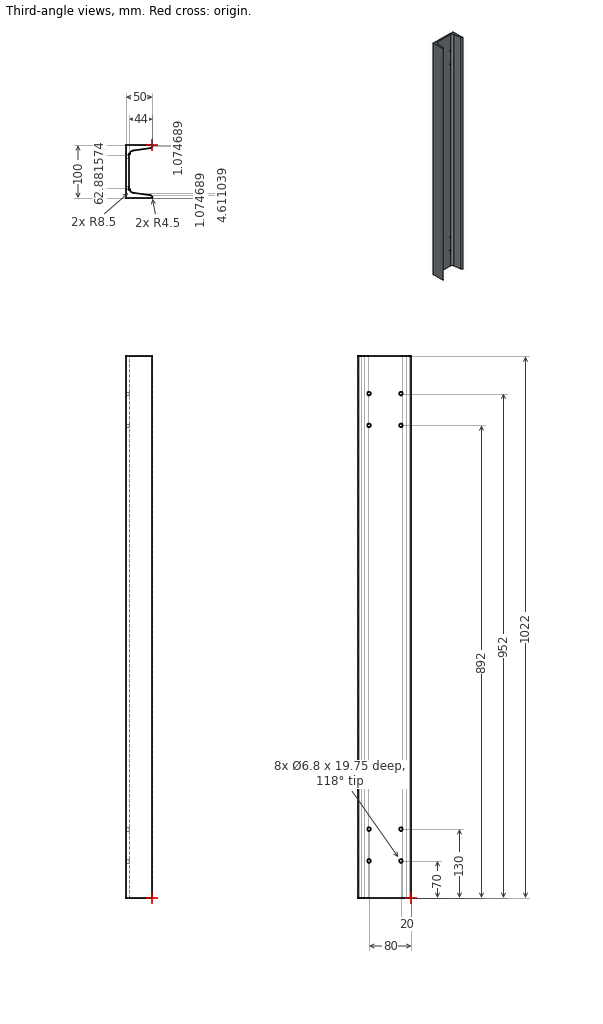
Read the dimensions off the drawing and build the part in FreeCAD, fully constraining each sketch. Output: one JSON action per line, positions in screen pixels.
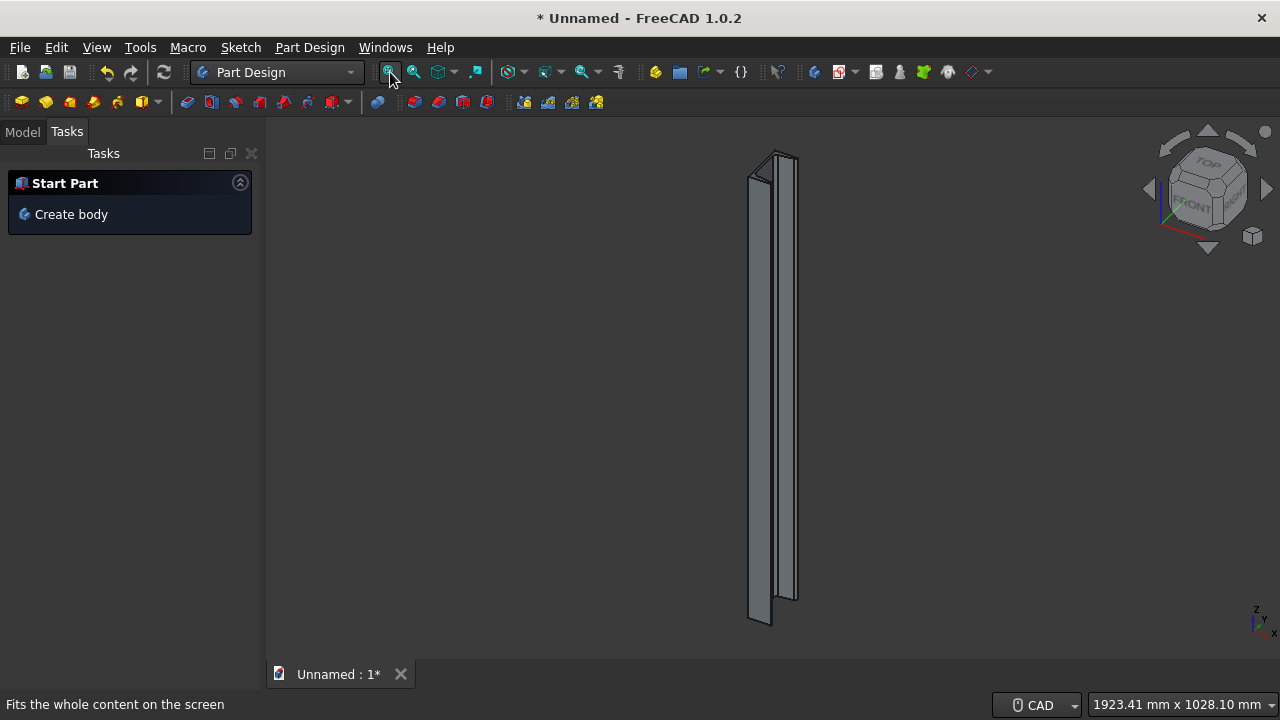
{"action": "key", "text": "6"}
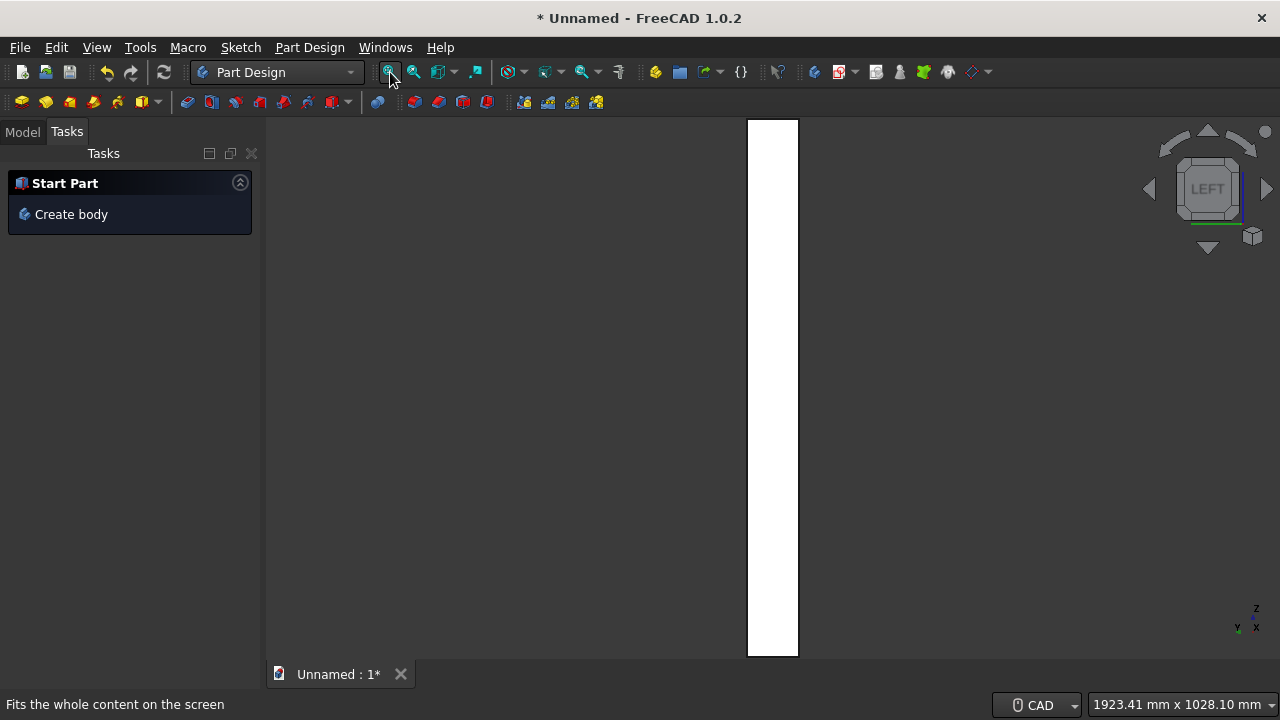
{"action": "left_click", "coordinate": [773, 156]}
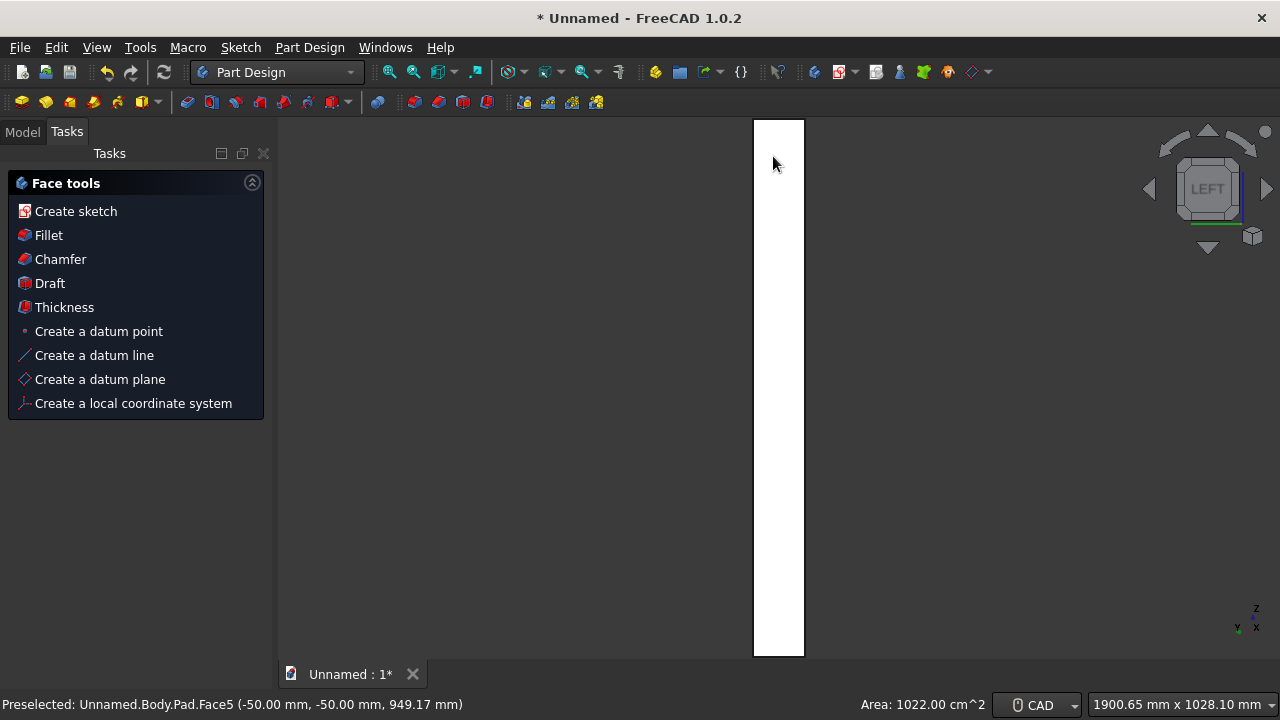
{"action": "left_click", "coordinate": [840, 72]}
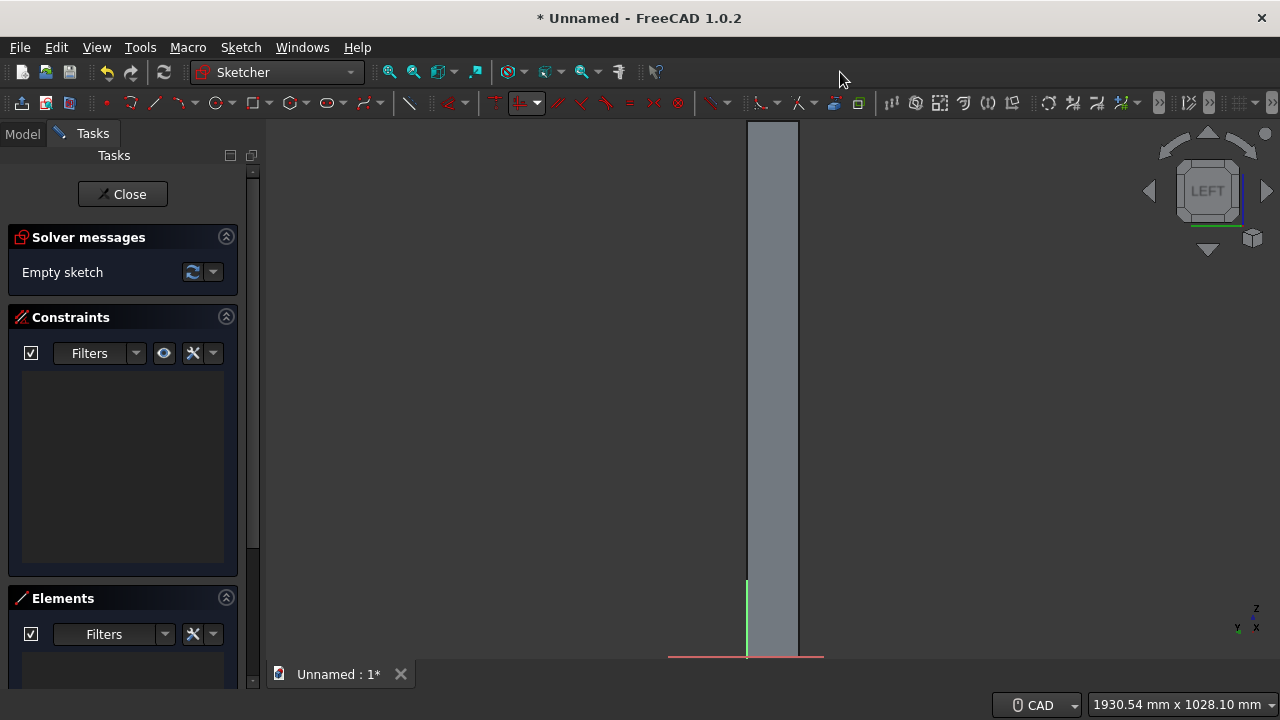
{"action": "scroll", "coordinate": [574, 353], "scroll_direction": "down", "scroll_amount": 2}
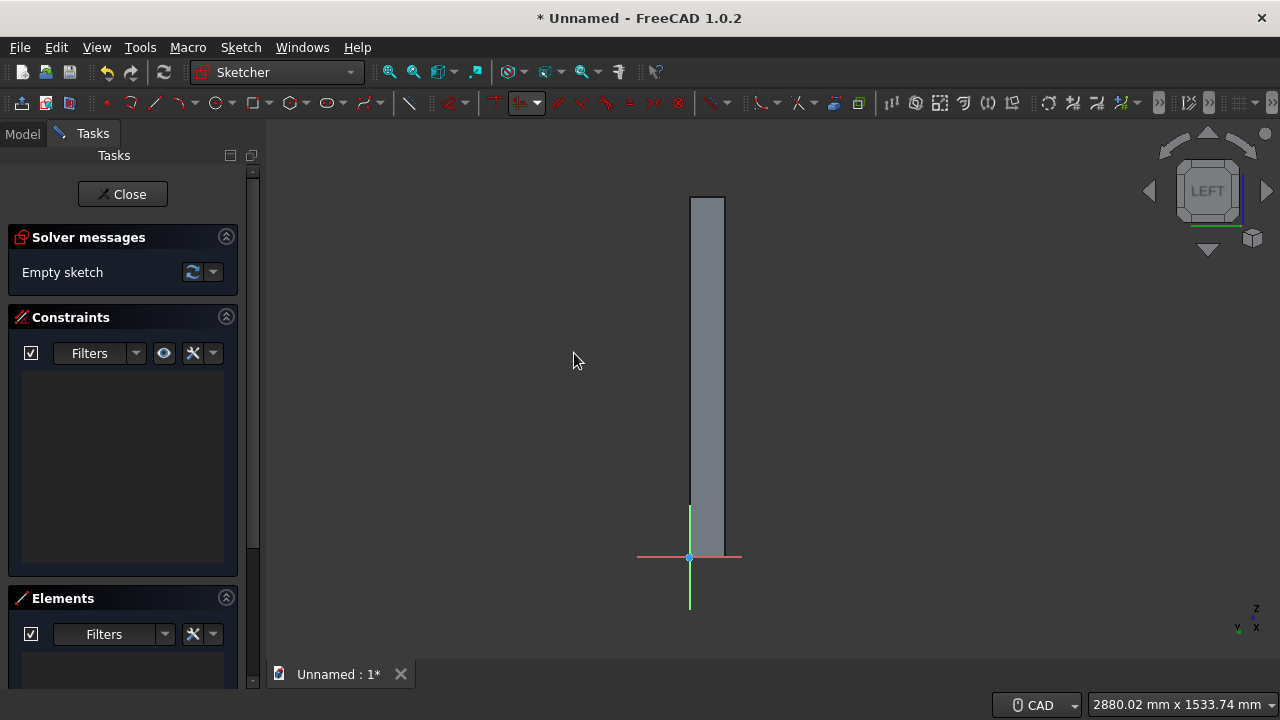
{"action": "left_click", "coordinate": [216, 104]}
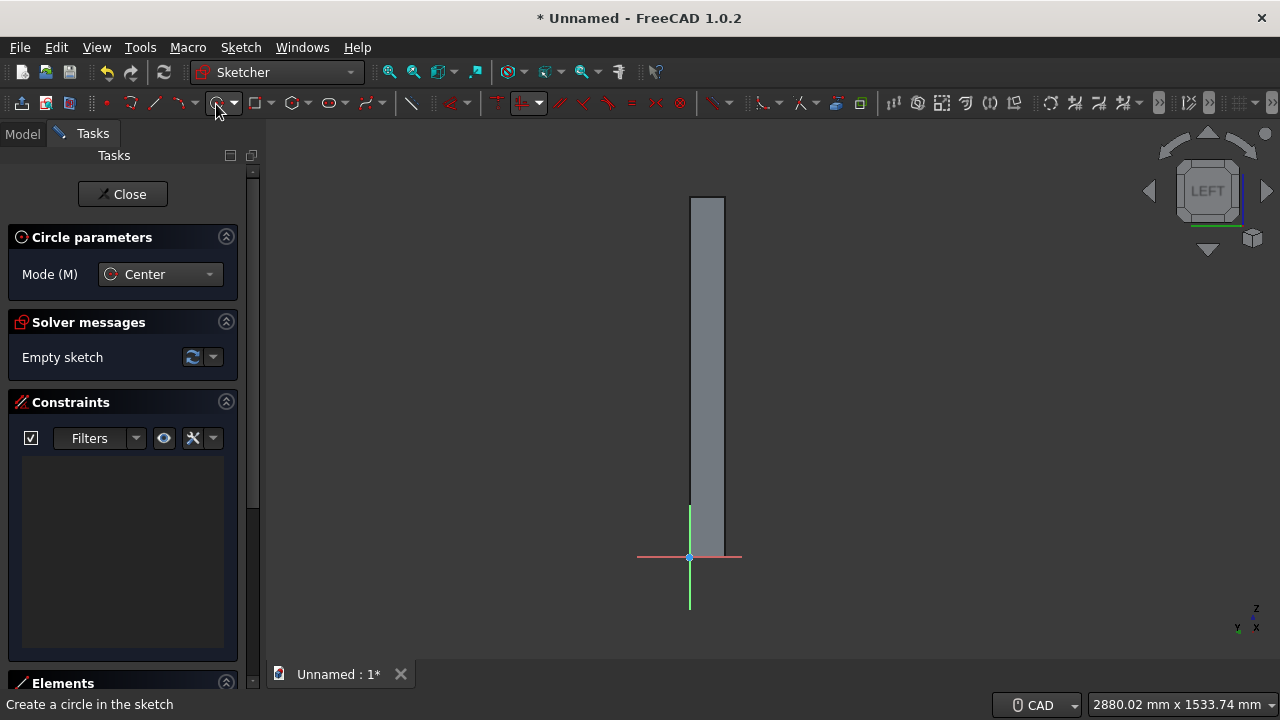
{"action": "scroll", "coordinate": [697, 533], "scroll_direction": "up", "scroll_amount": 15}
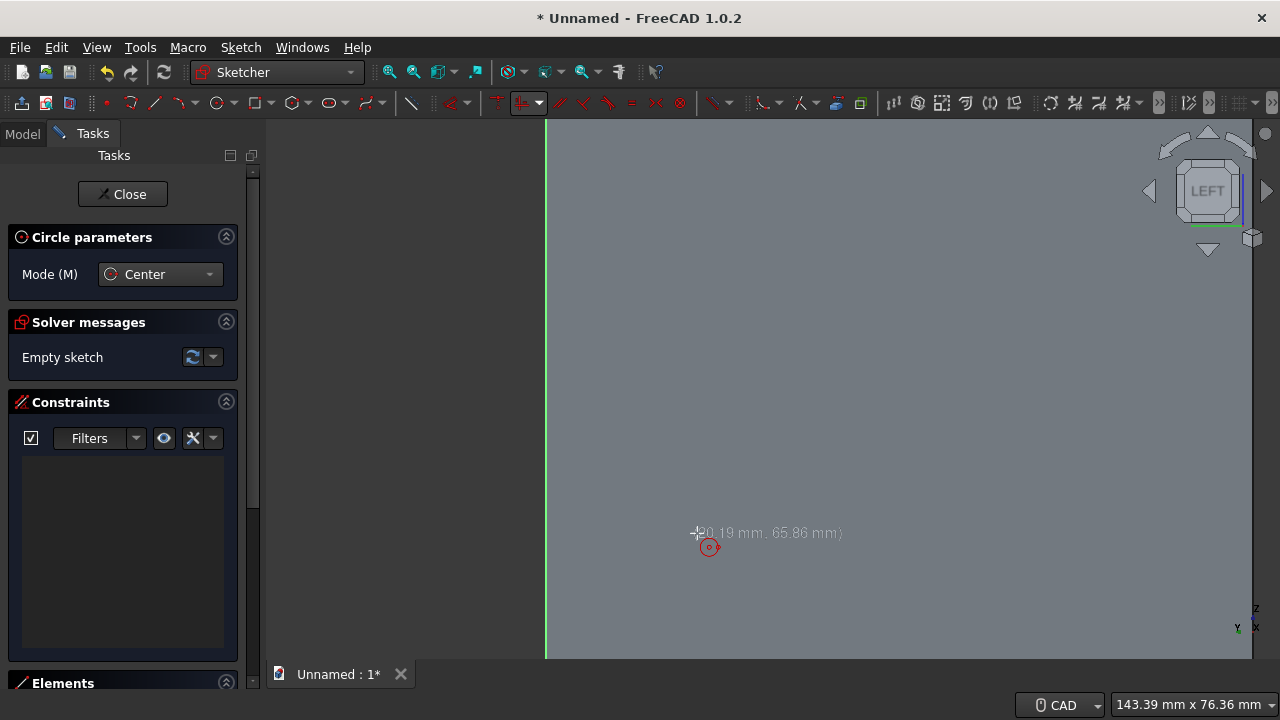
{"action": "scroll", "coordinate": [697, 534], "scroll_direction": "down", "scroll_amount": 15}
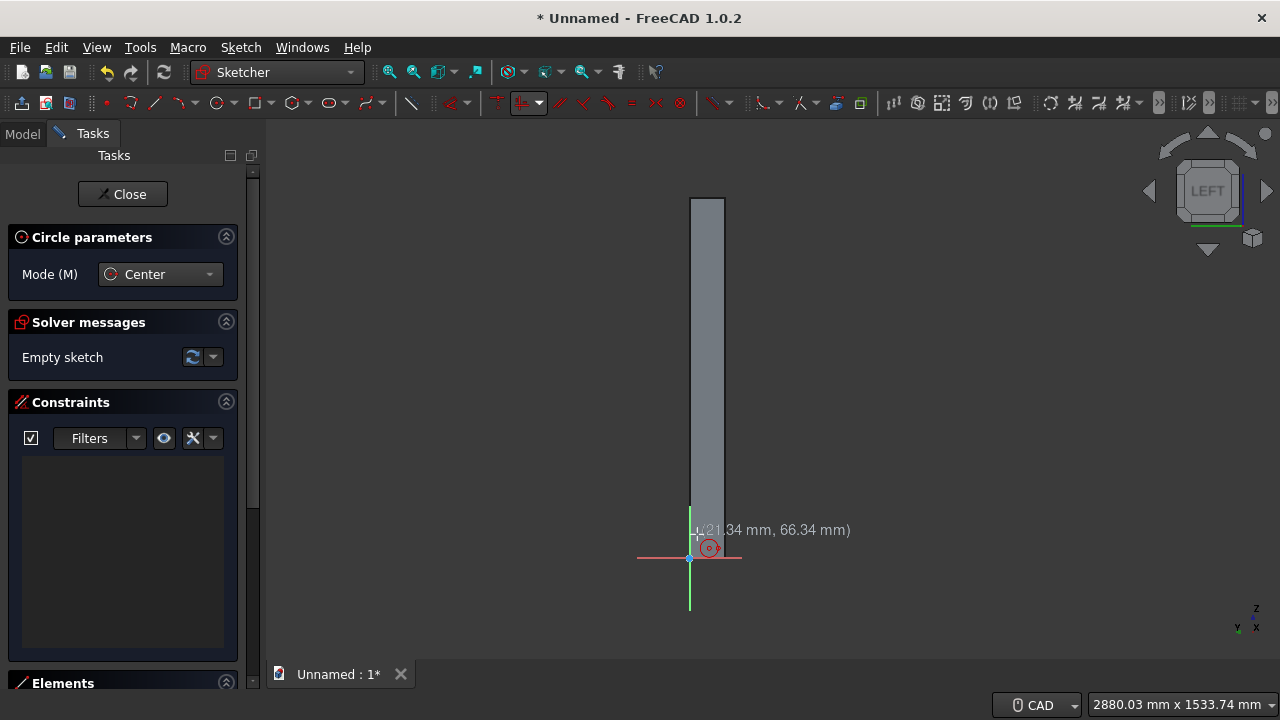
{"action": "scroll", "coordinate": [697, 533], "scroll_direction": "up", "scroll_amount": 5}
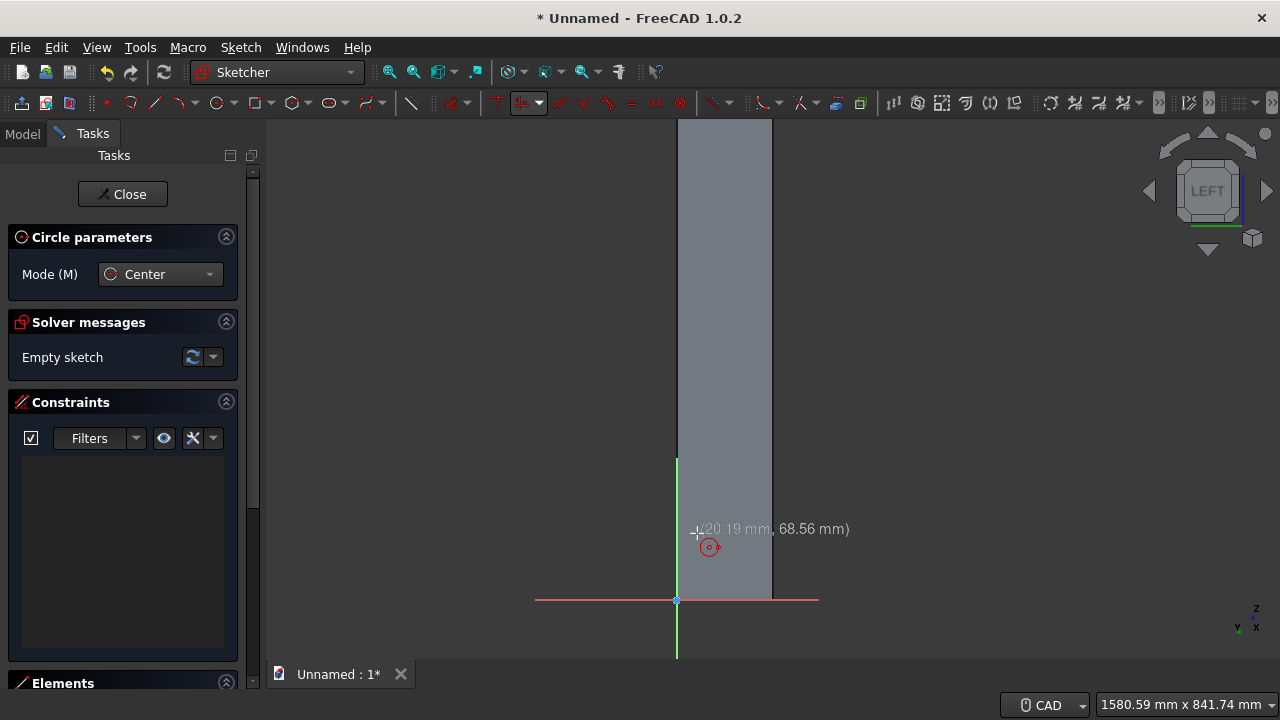
{"action": "left_click", "coordinate": [696, 533]}
{"action": "mouse_move", "coordinate": [698, 531]}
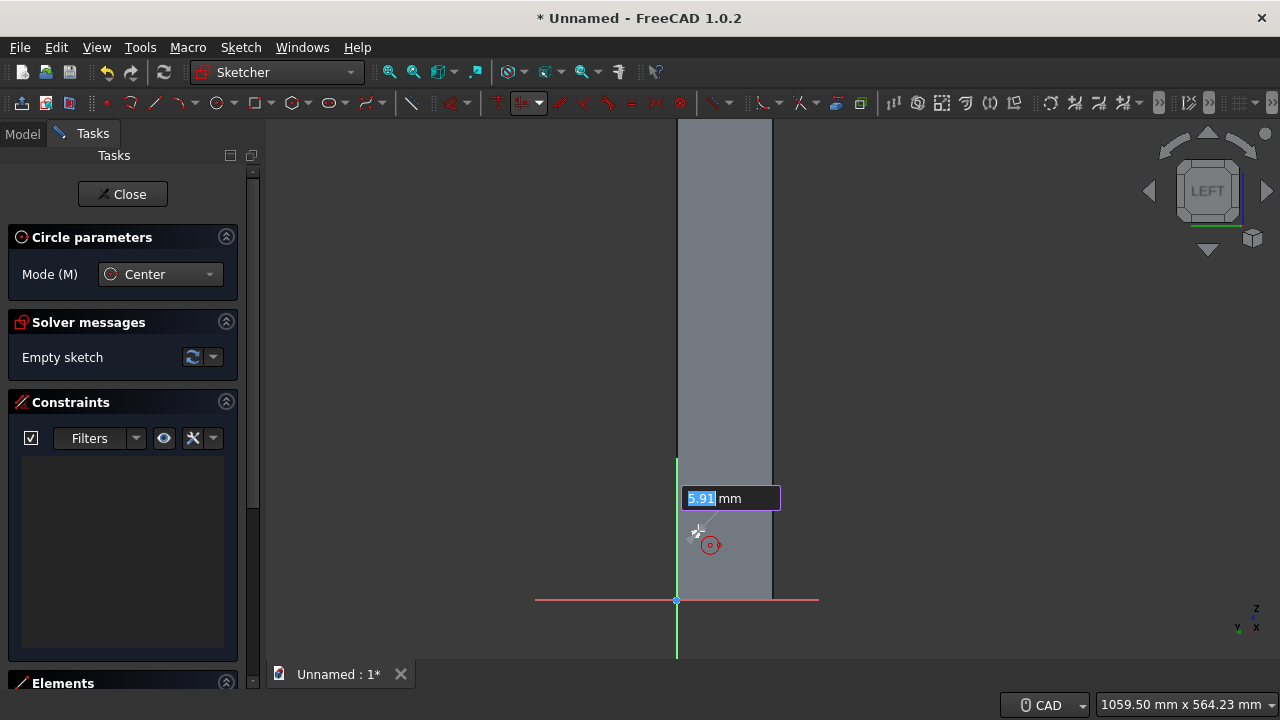
{"action": "type", "text": "6.8"}
{"action": "key", "text": "Return"}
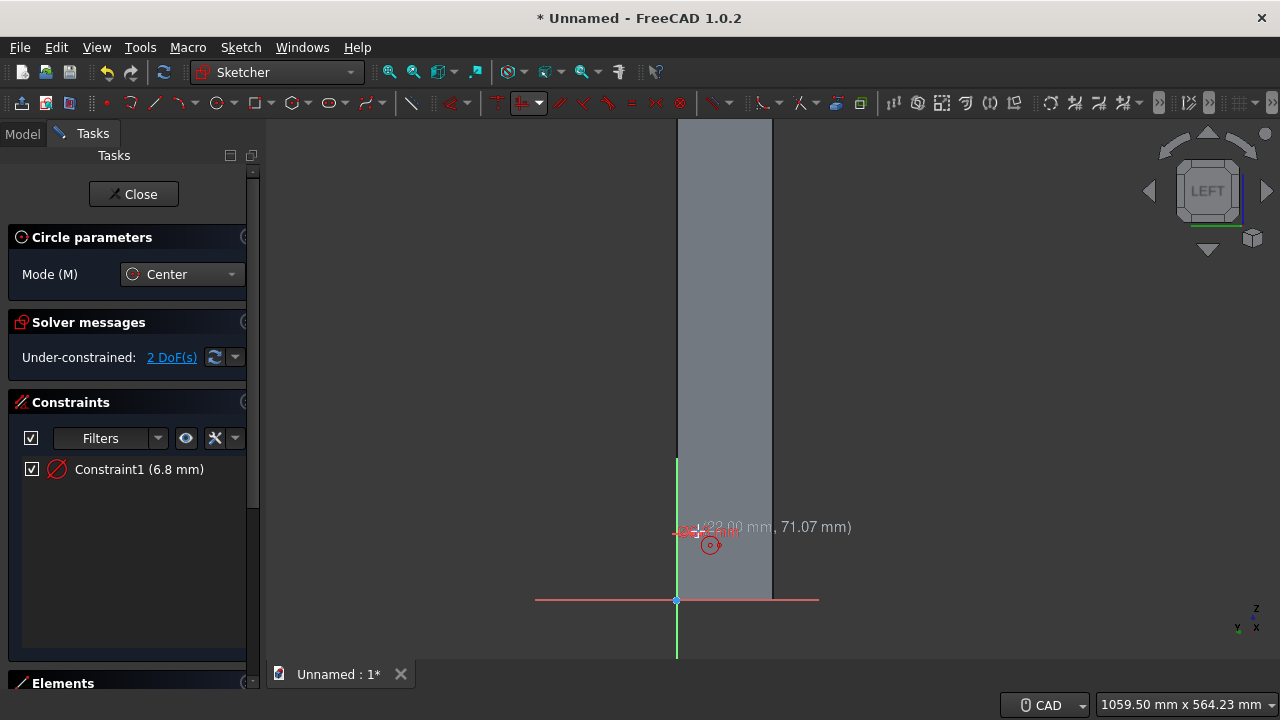
{"action": "scroll", "coordinate": [696, 476], "scroll_direction": "up", "scroll_amount": 10}